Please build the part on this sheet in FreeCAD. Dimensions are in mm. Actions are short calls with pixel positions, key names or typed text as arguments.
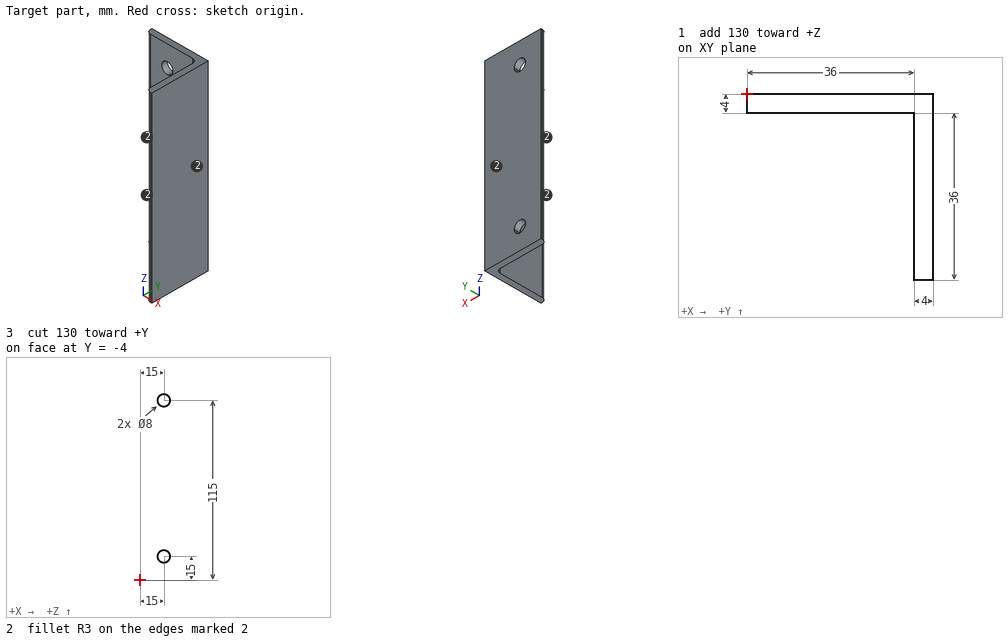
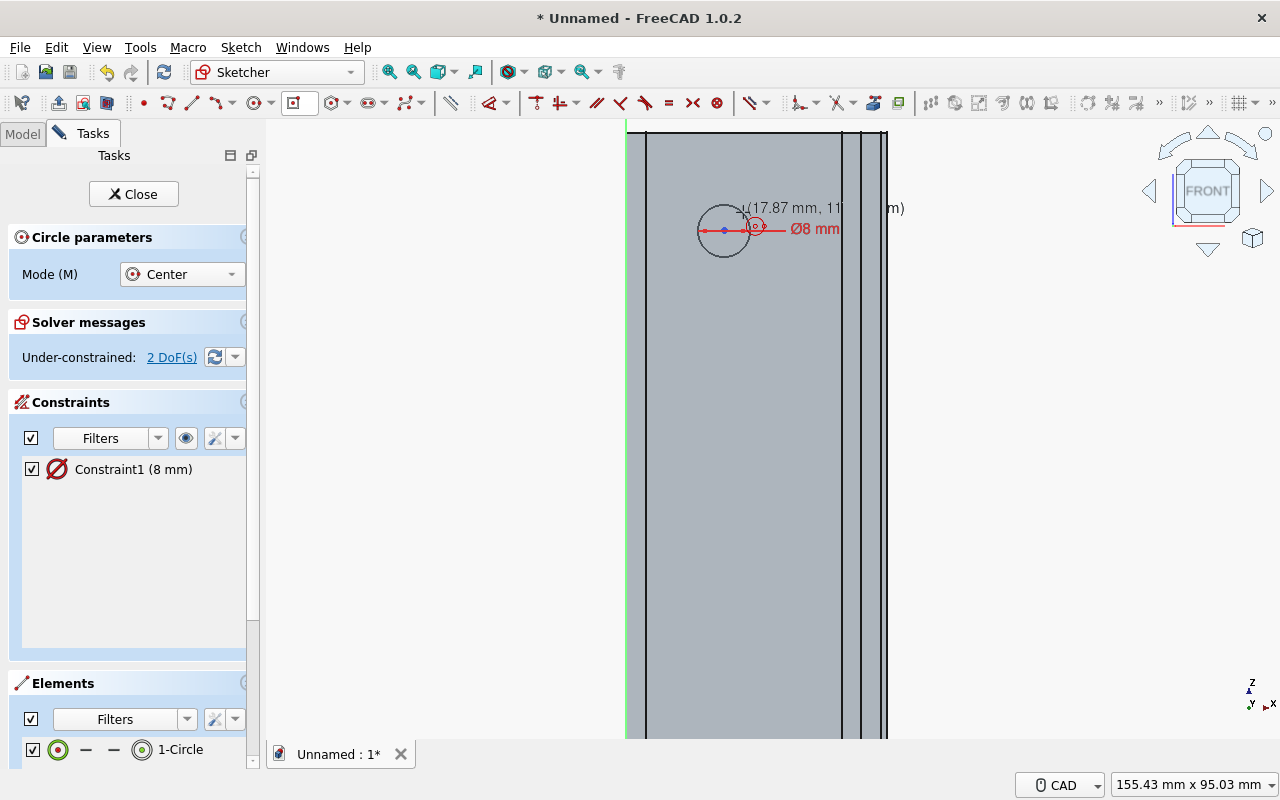
scroll(724, 230, down, 3)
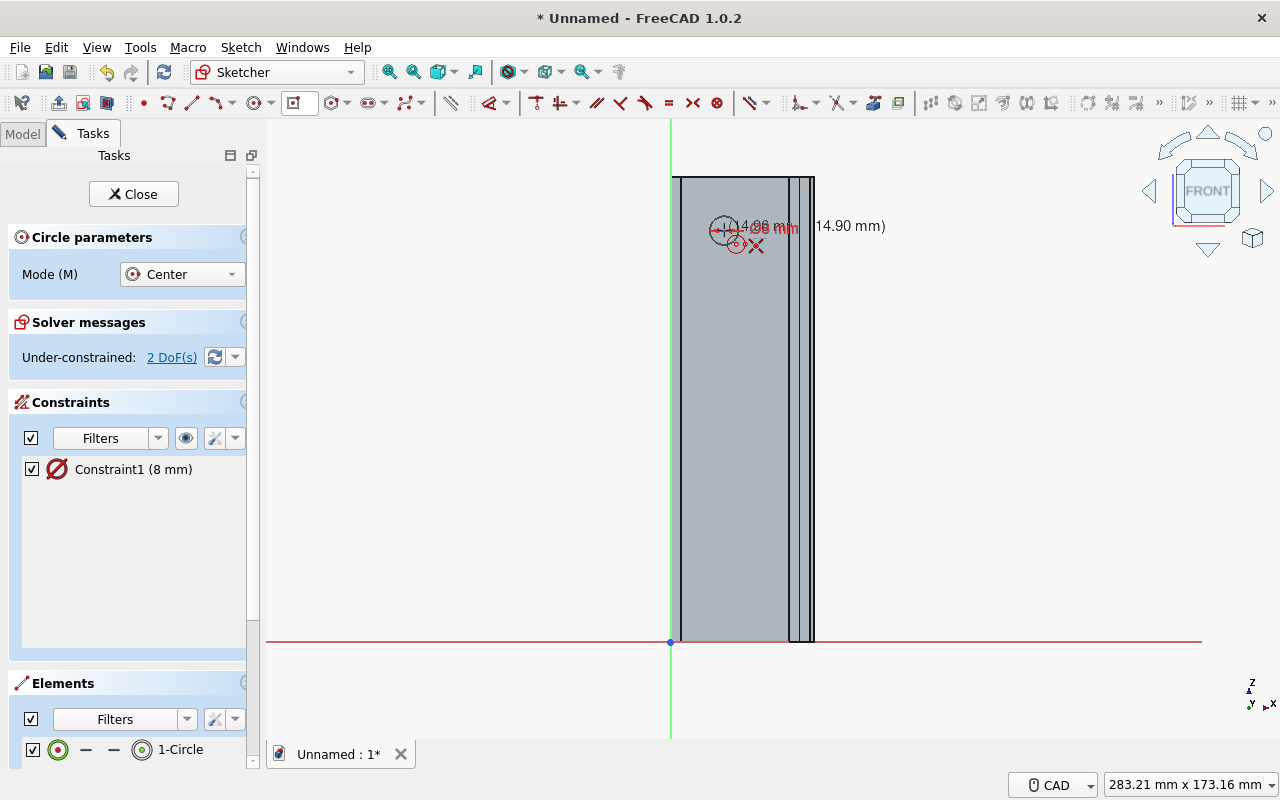
scroll(724, 588, up, 3)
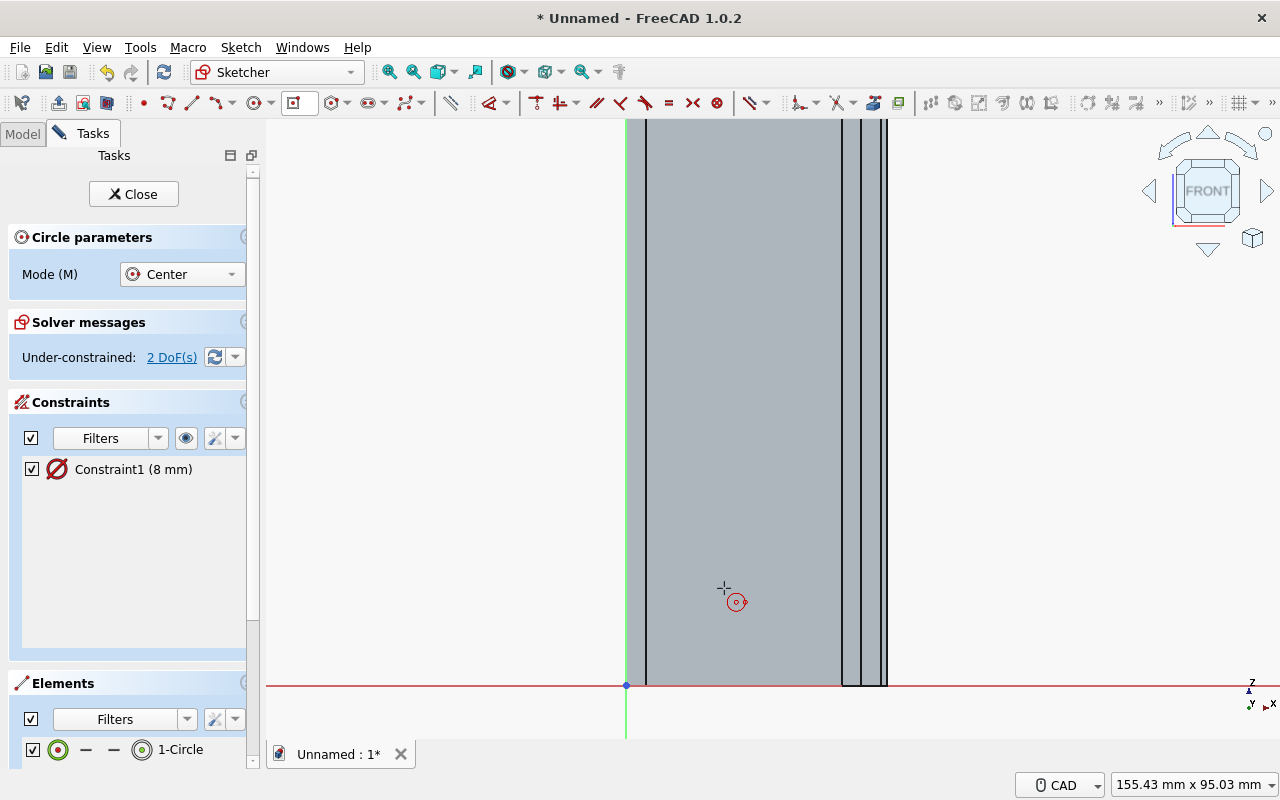
click(724, 588)
move(743, 570)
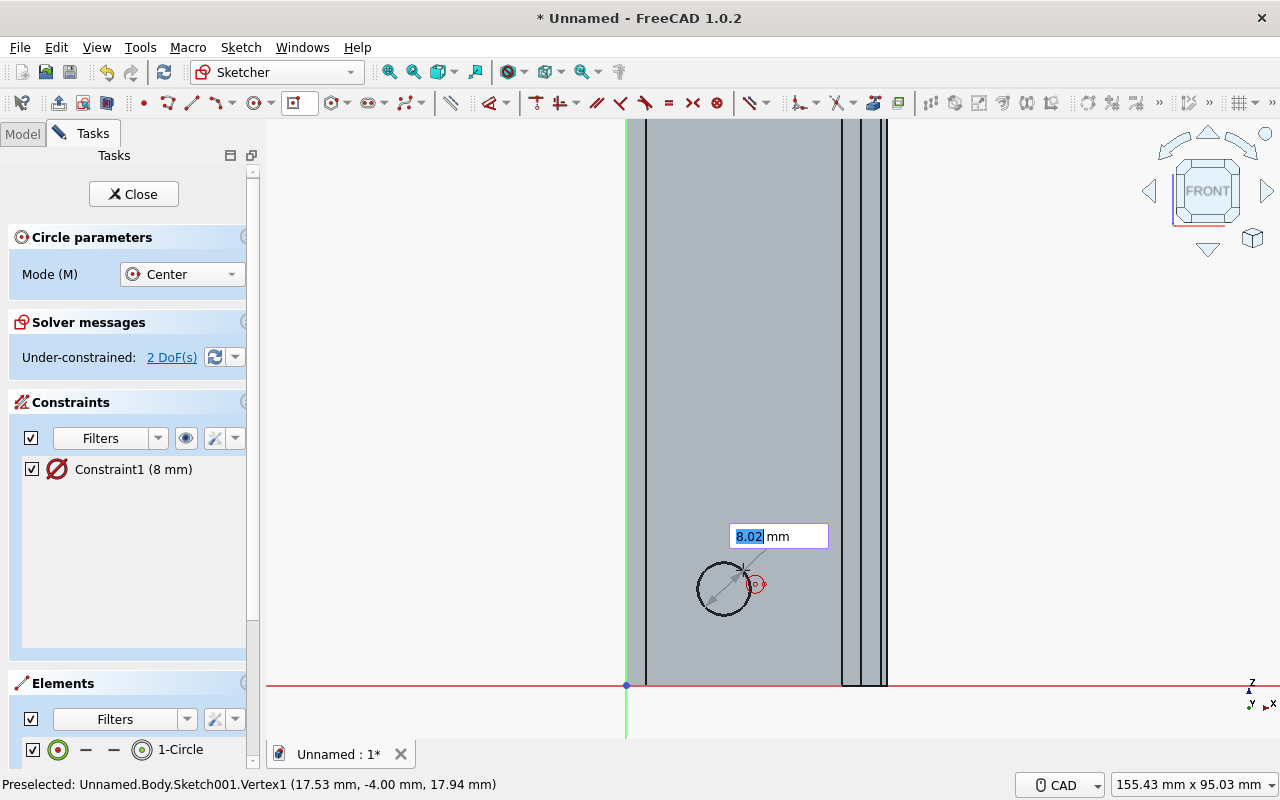
text(8)
key(Return)
key(Escape)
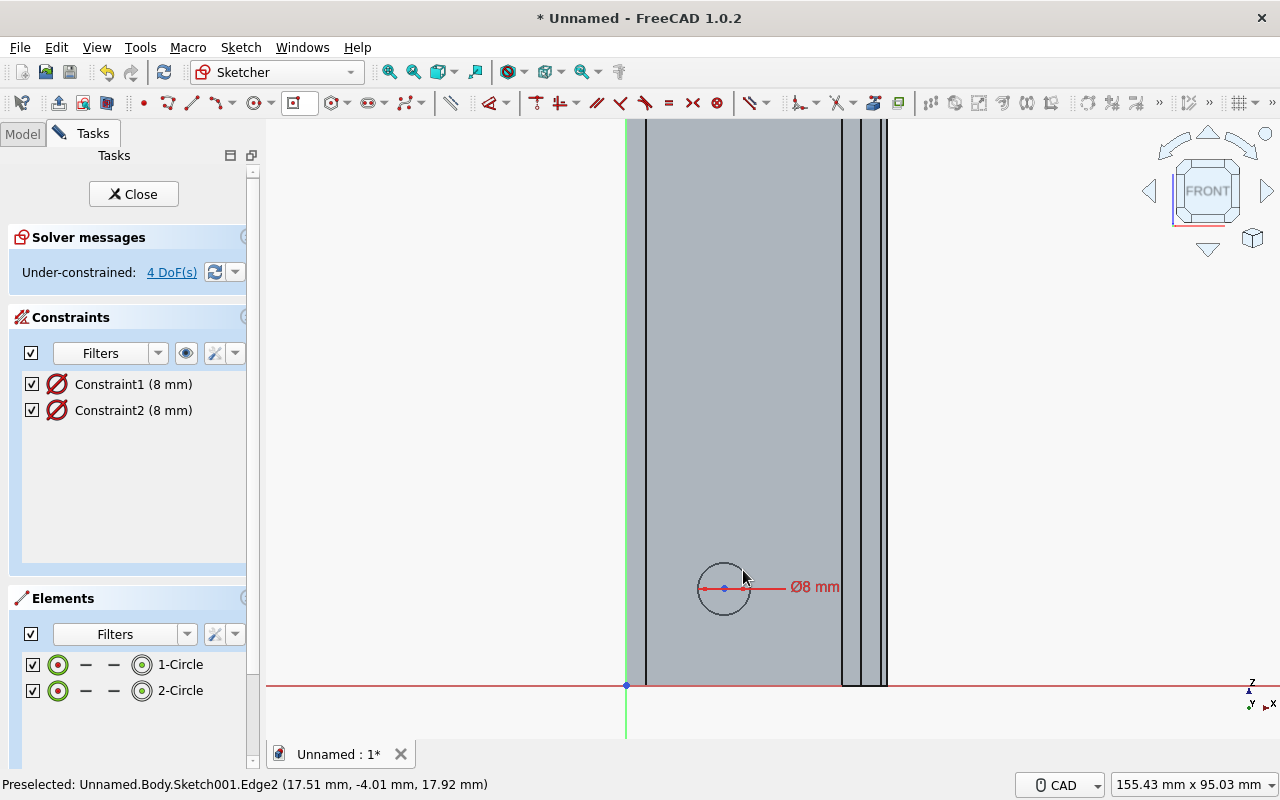
click(490, 104)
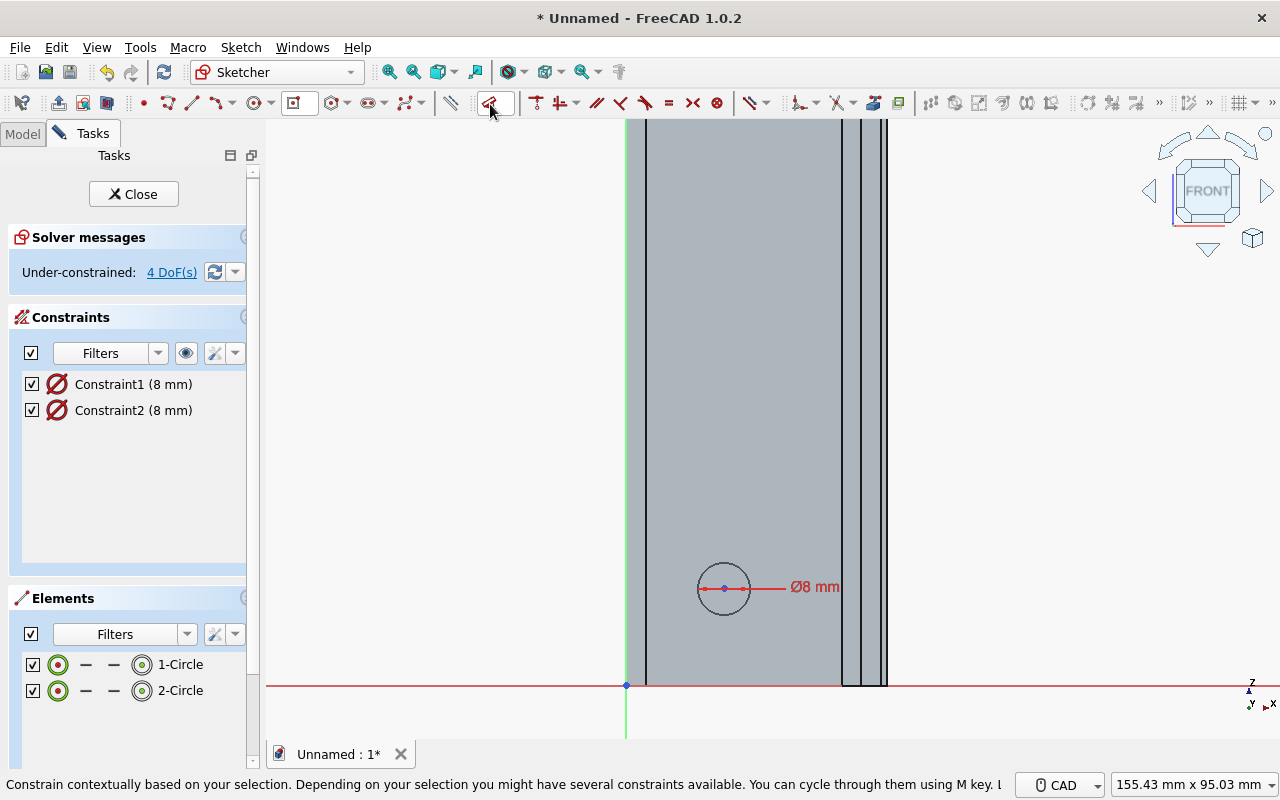
scroll(724, 589, down, 3)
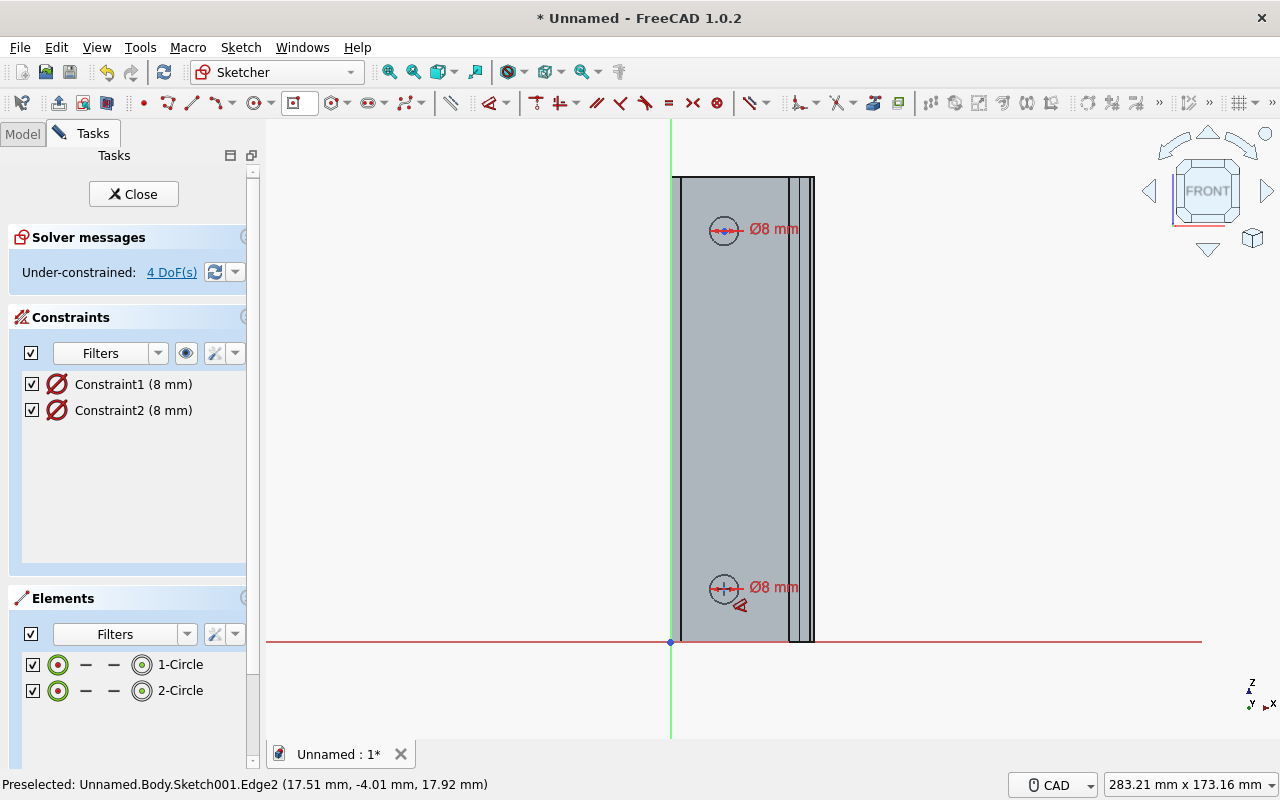
click(724, 231)
click(697, 676)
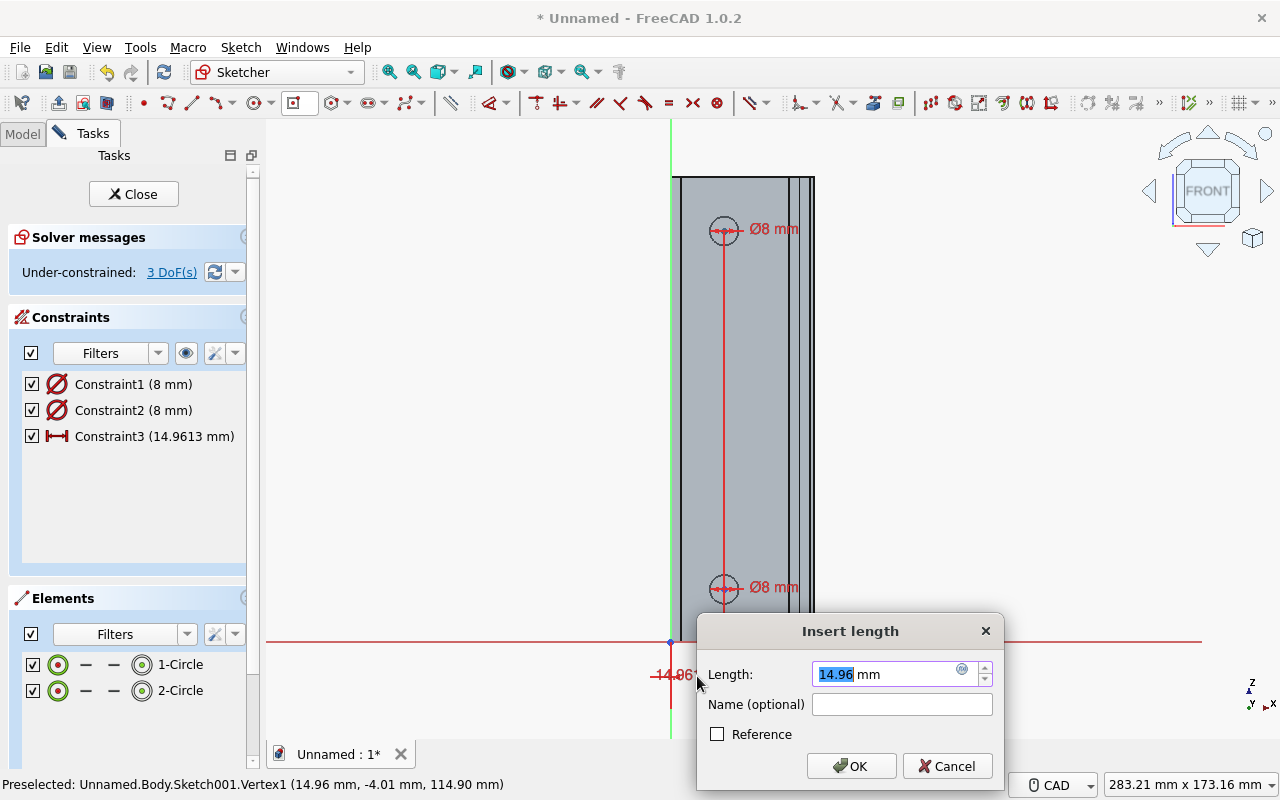
text(15)
key(Return)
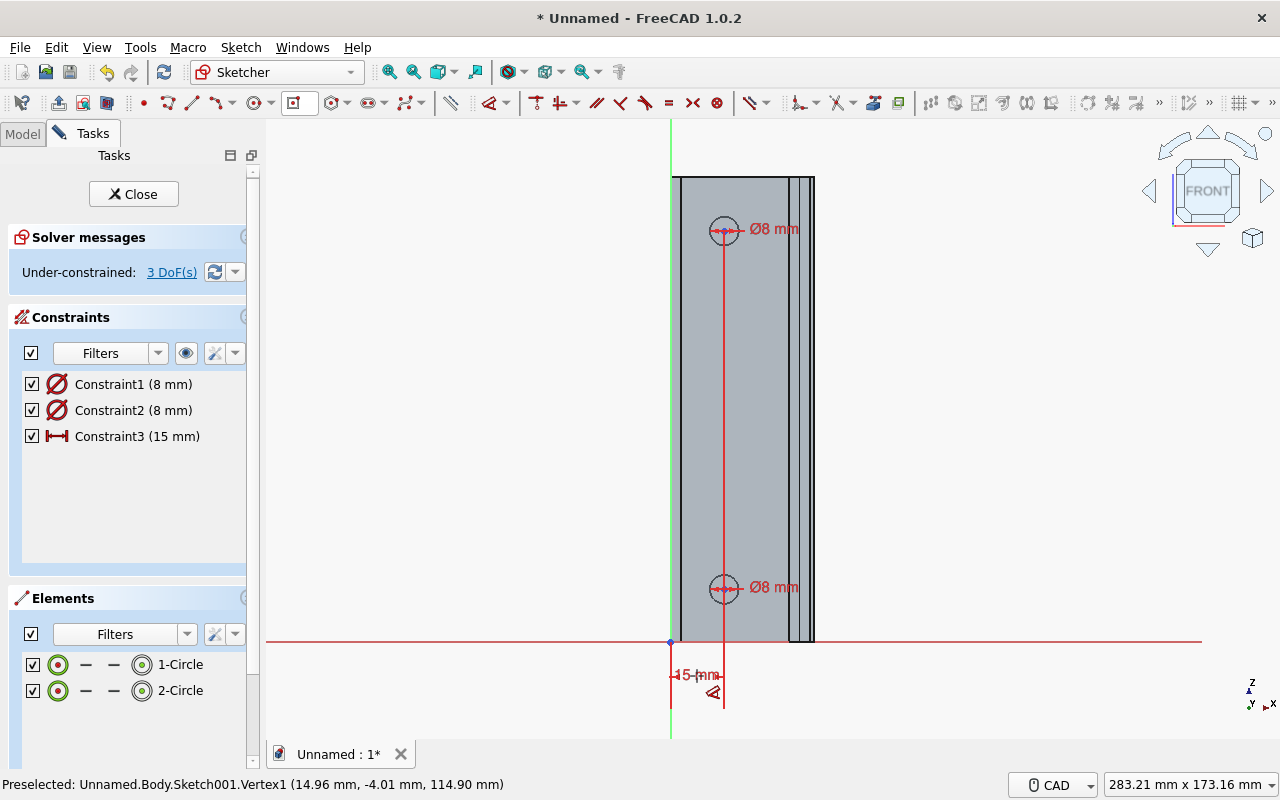
click(724, 589)
click(697, 555)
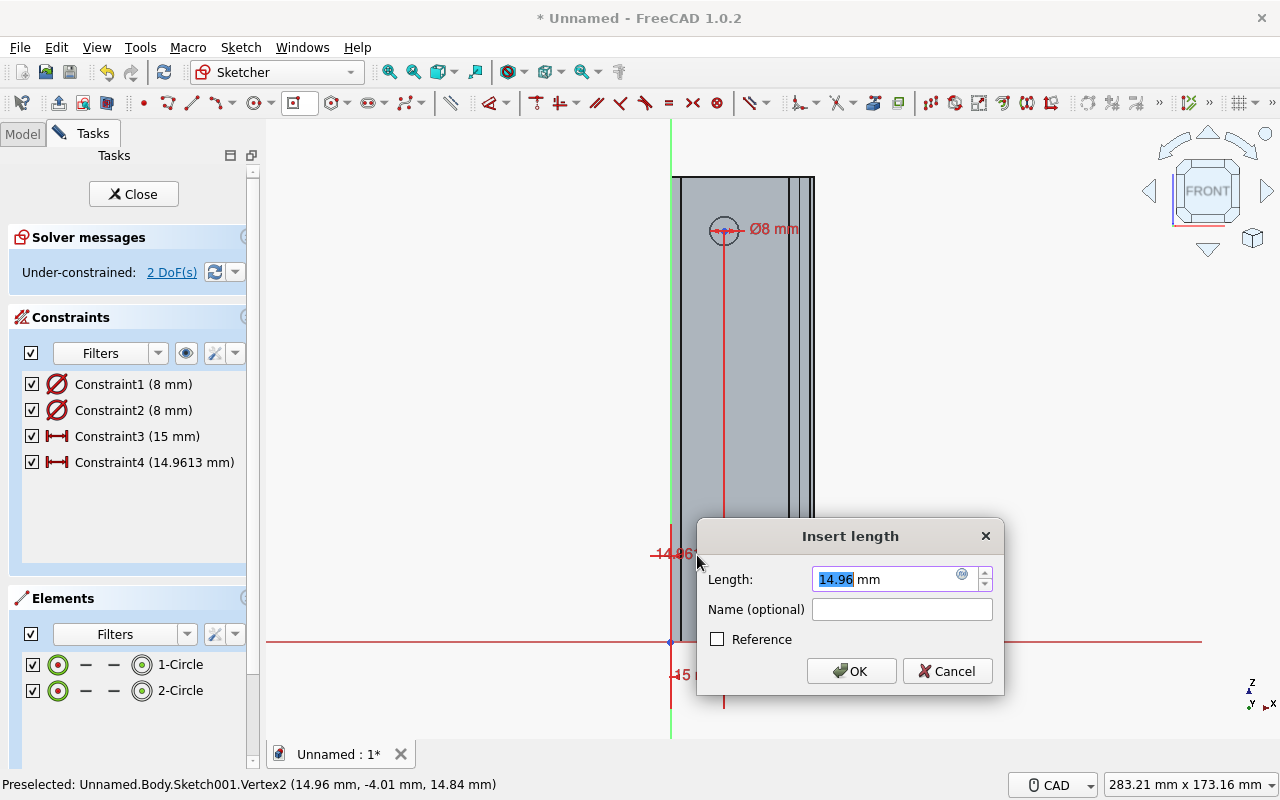
text(15)
key(Return)